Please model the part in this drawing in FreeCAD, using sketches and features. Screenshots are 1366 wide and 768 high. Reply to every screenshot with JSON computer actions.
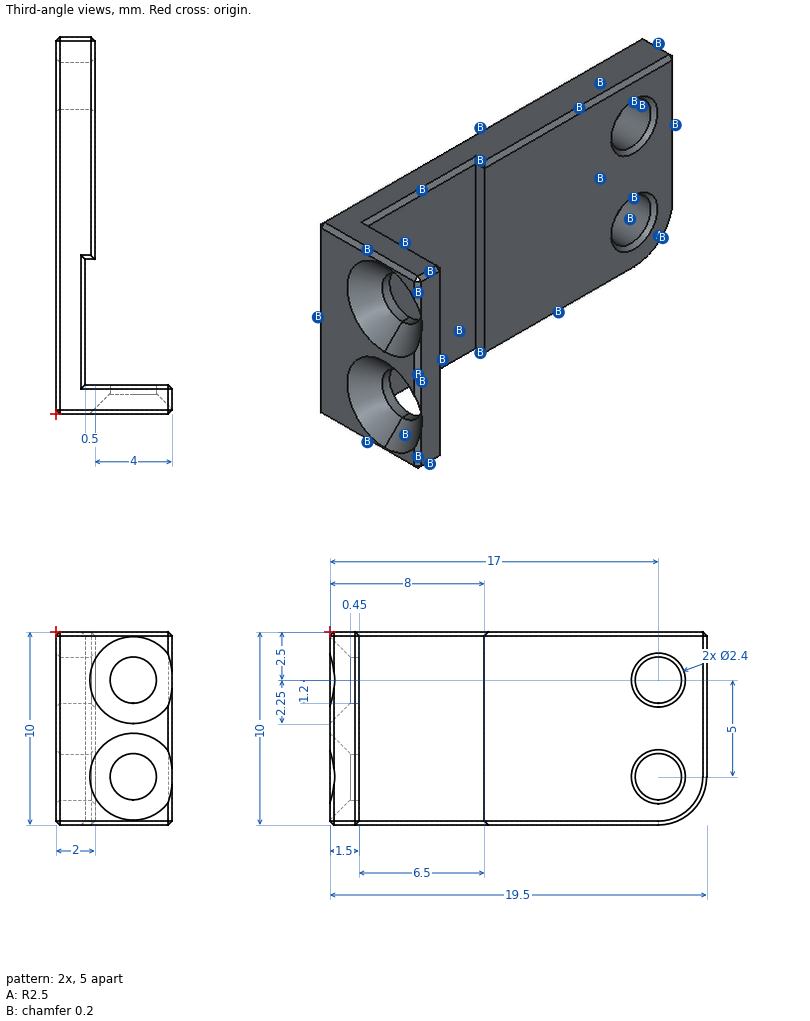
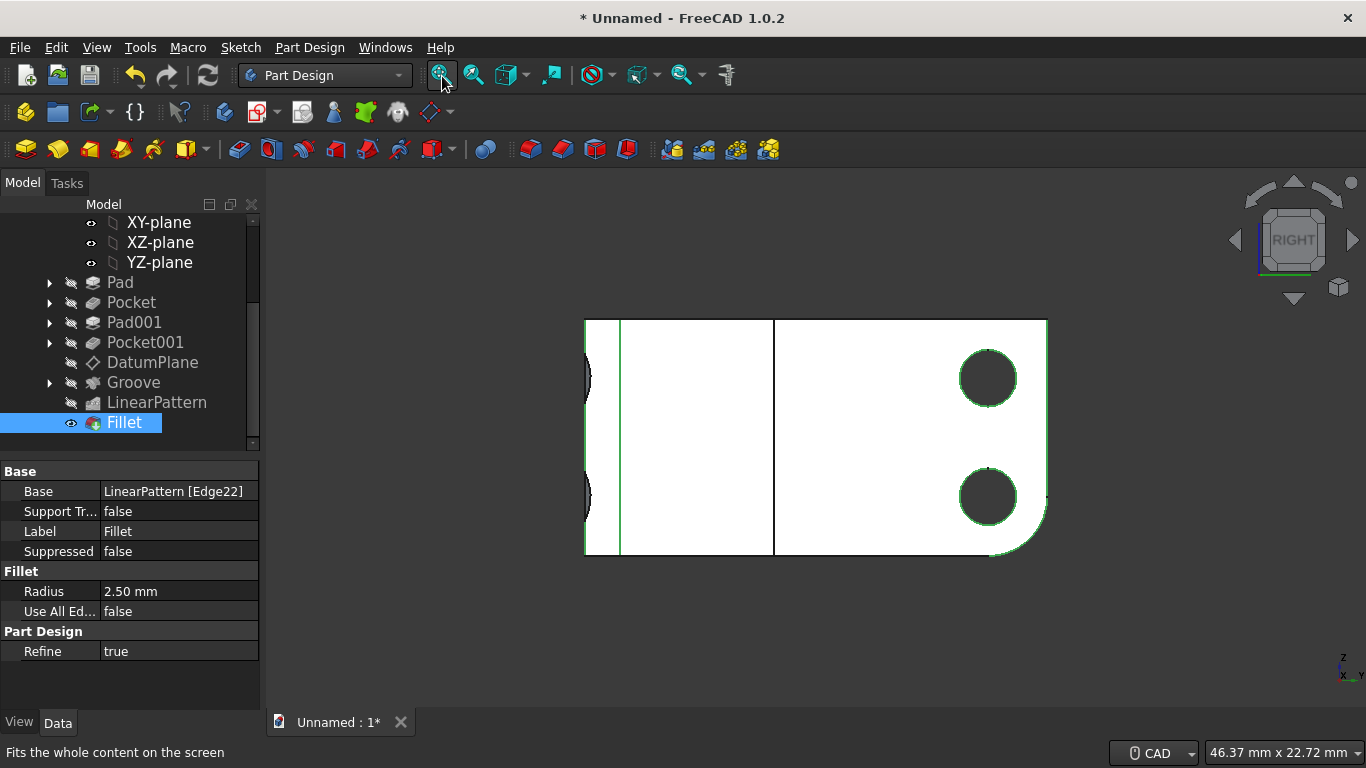
{"action": "left_click", "coordinate": [602, 555], "text": "ctrl"}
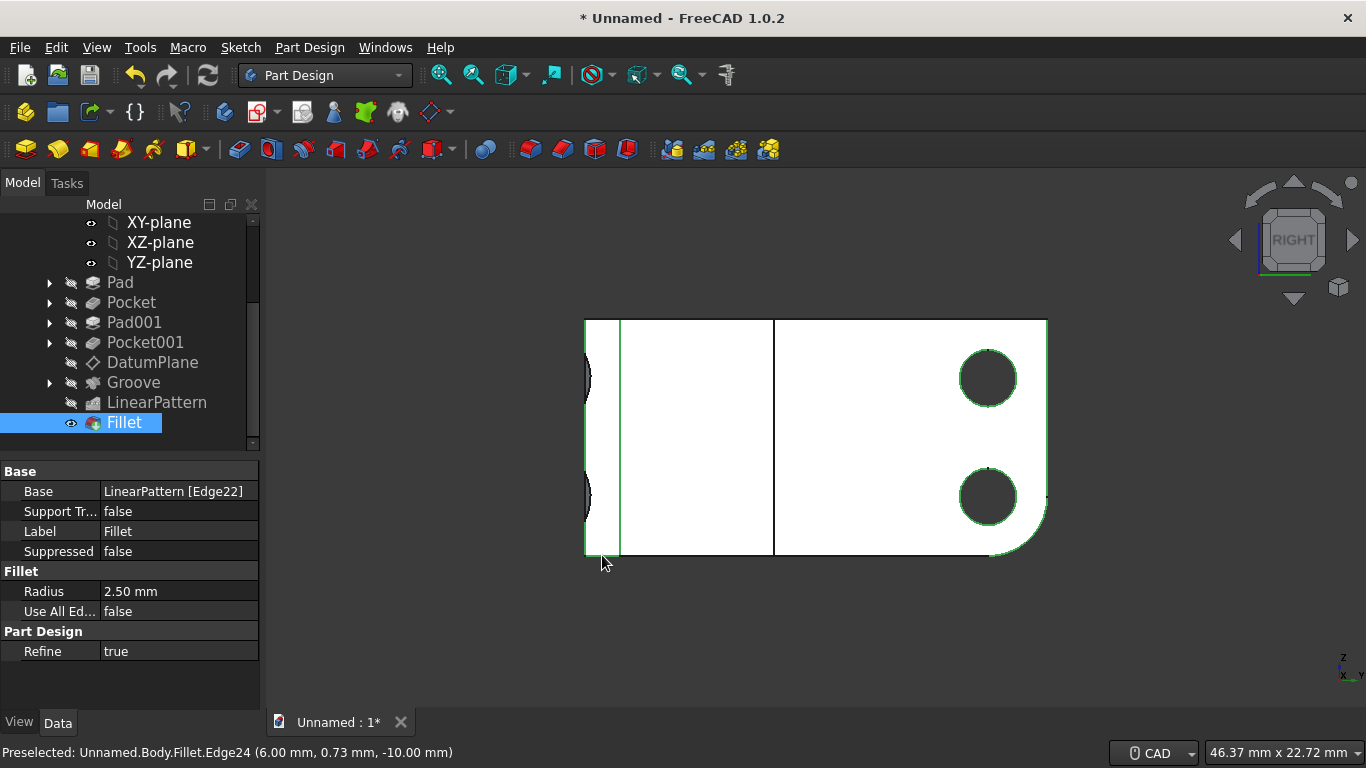
{"action": "left_click", "coordinate": [881, 555], "text": "ctrl"}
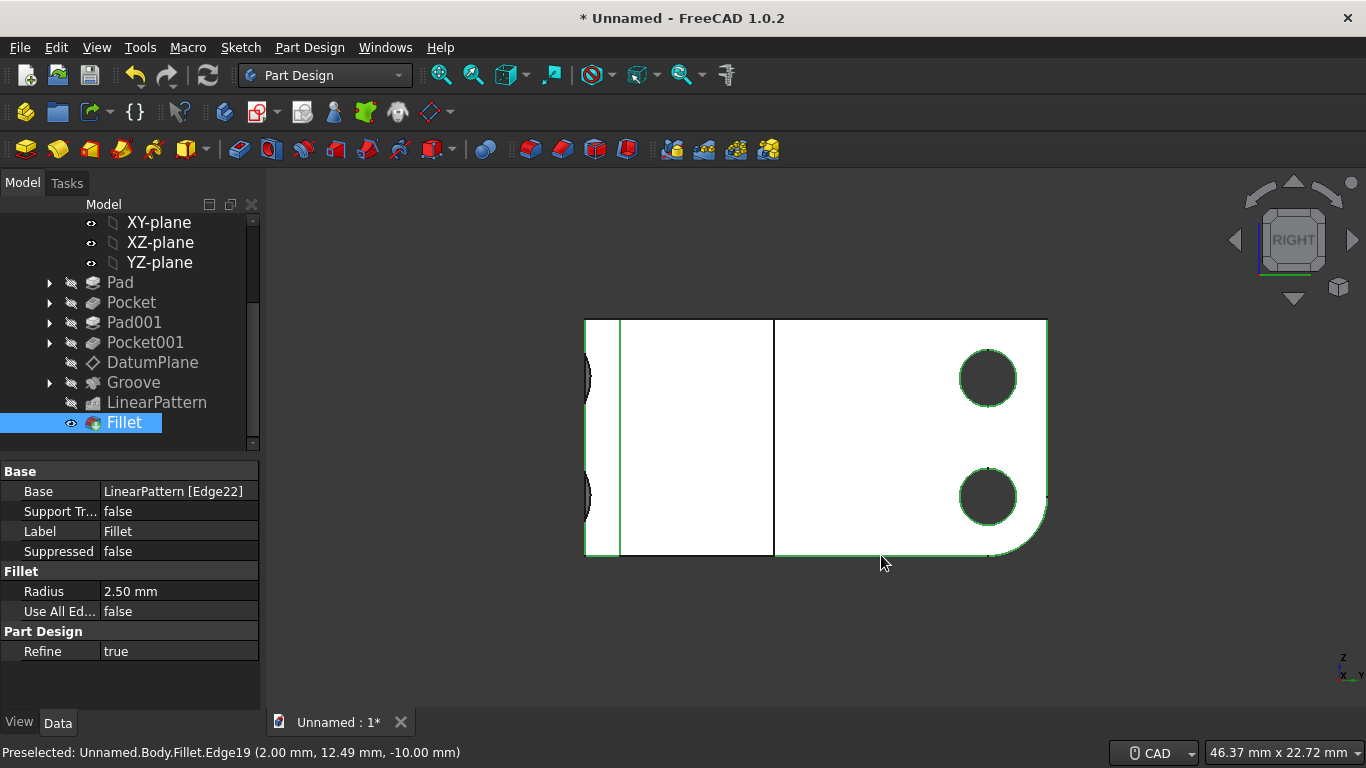
{"action": "left_click", "coordinate": [697, 555], "text": "ctrl"}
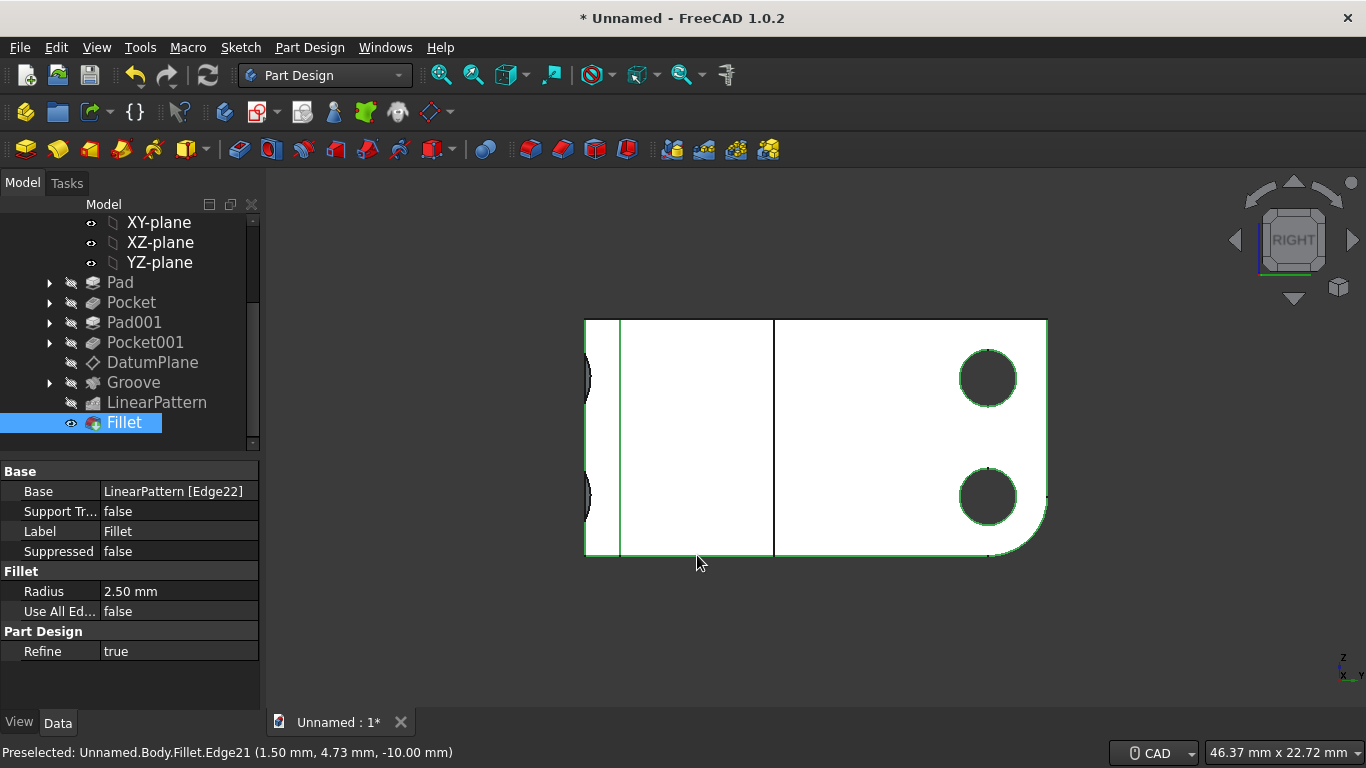
{"action": "key", "text": "5"}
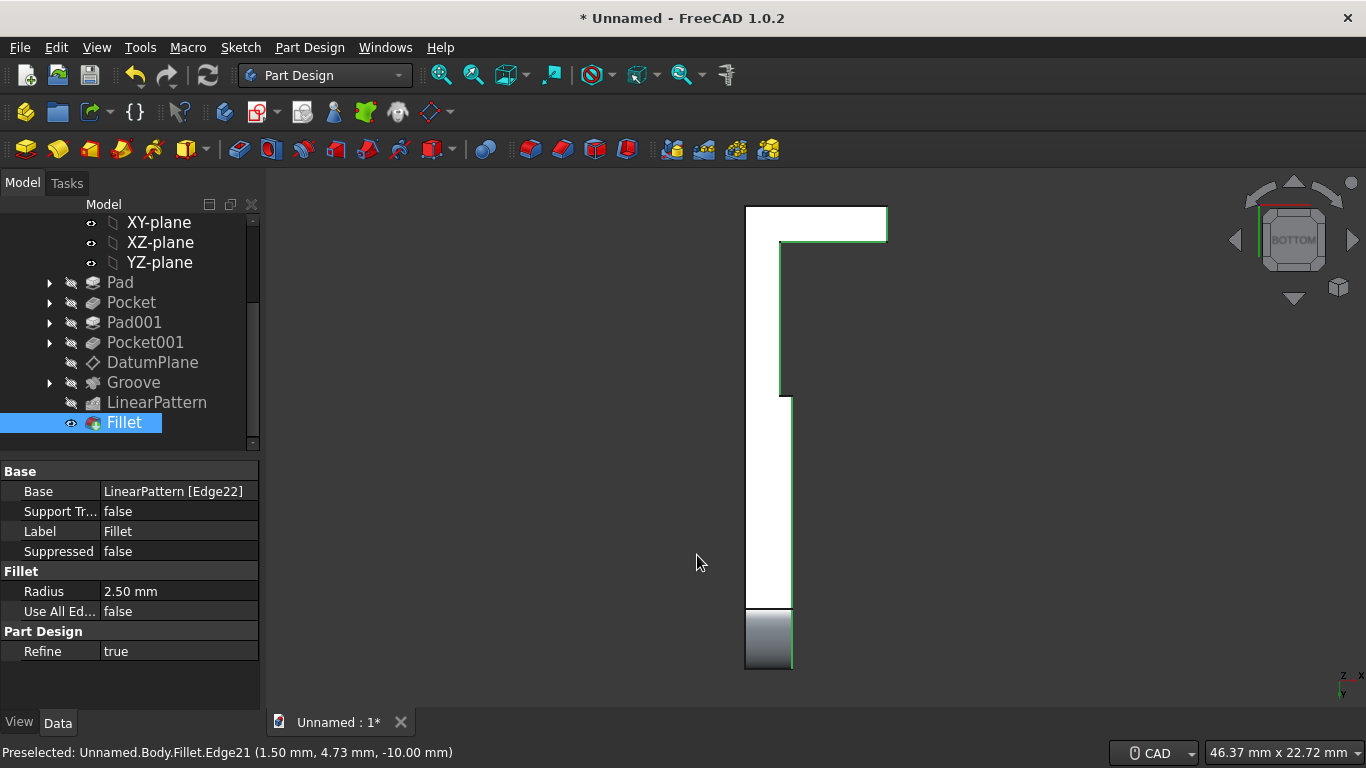
{"action": "left_click", "coordinate": [816, 205], "text": "ctrl"}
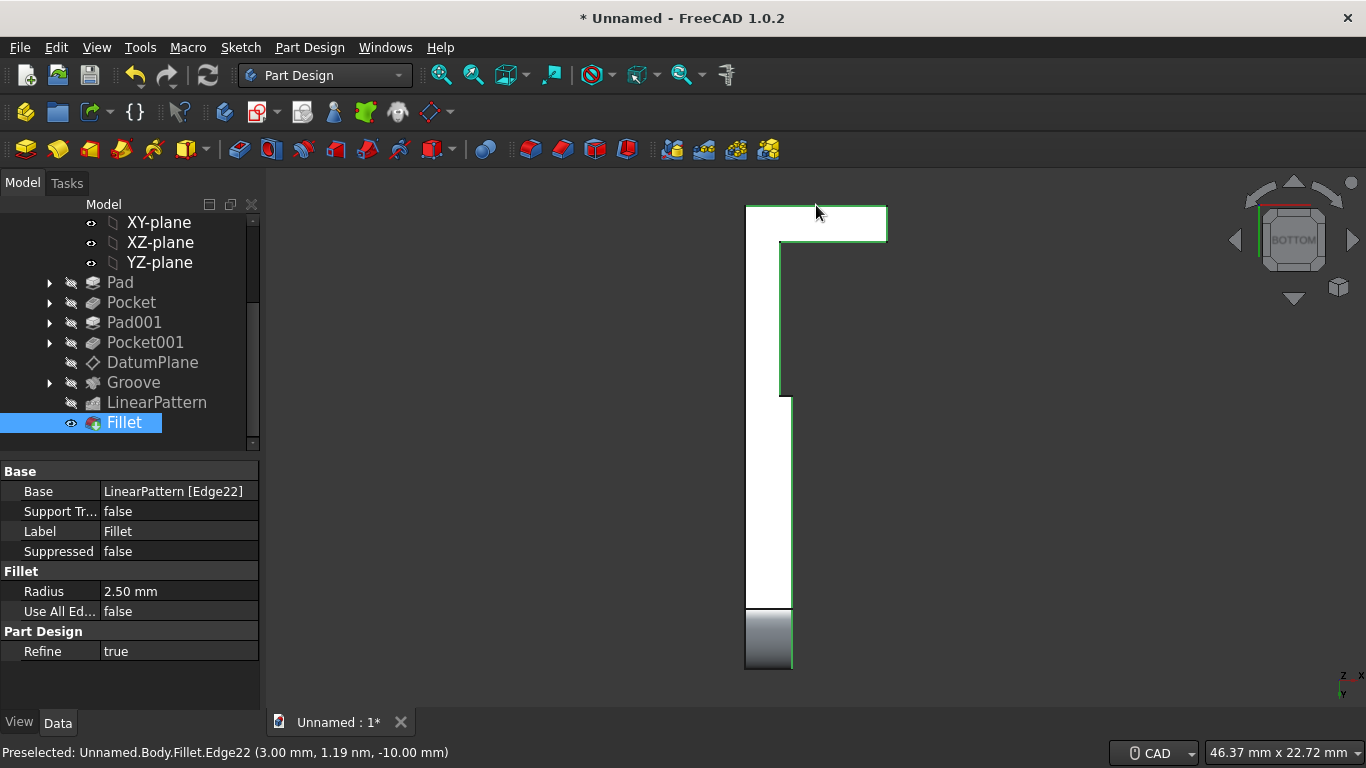
{"action": "key", "text": "4"}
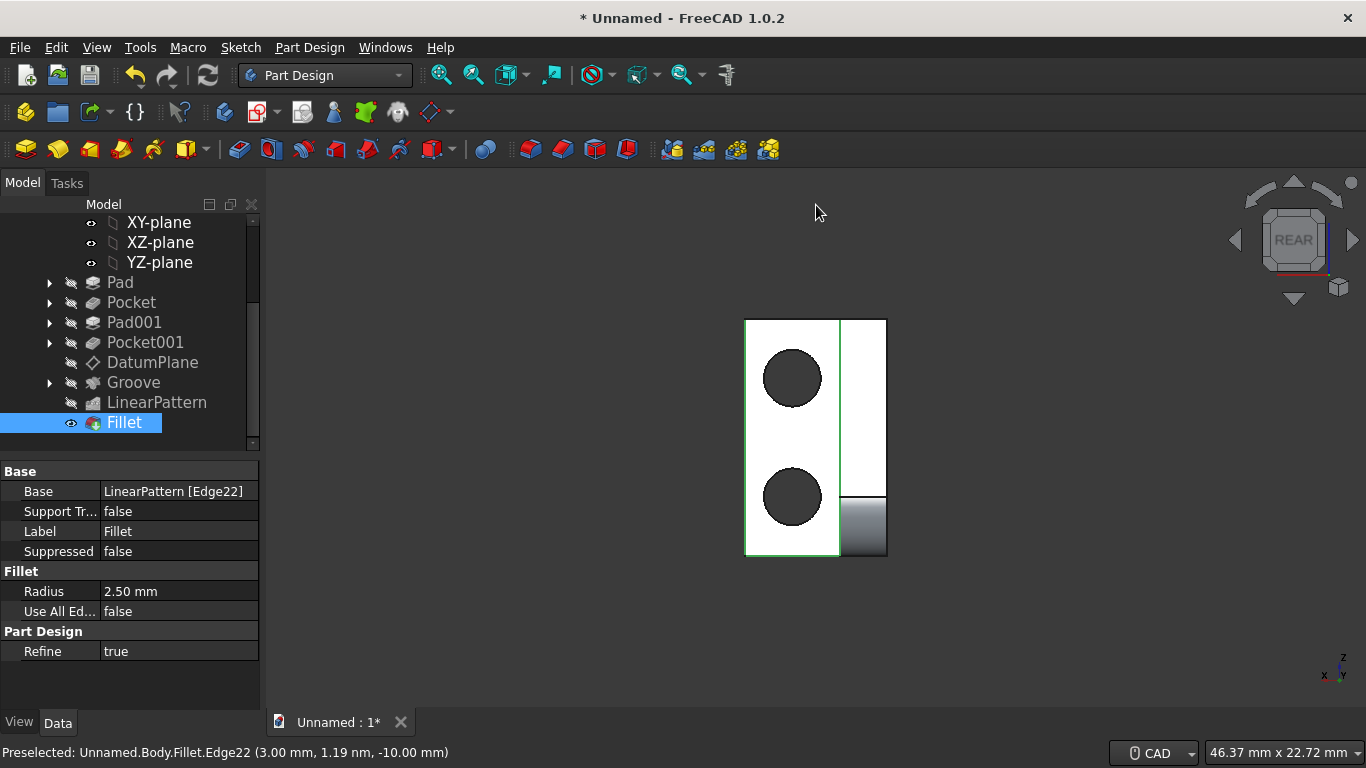
{"action": "left_click", "coordinate": [442, 76]}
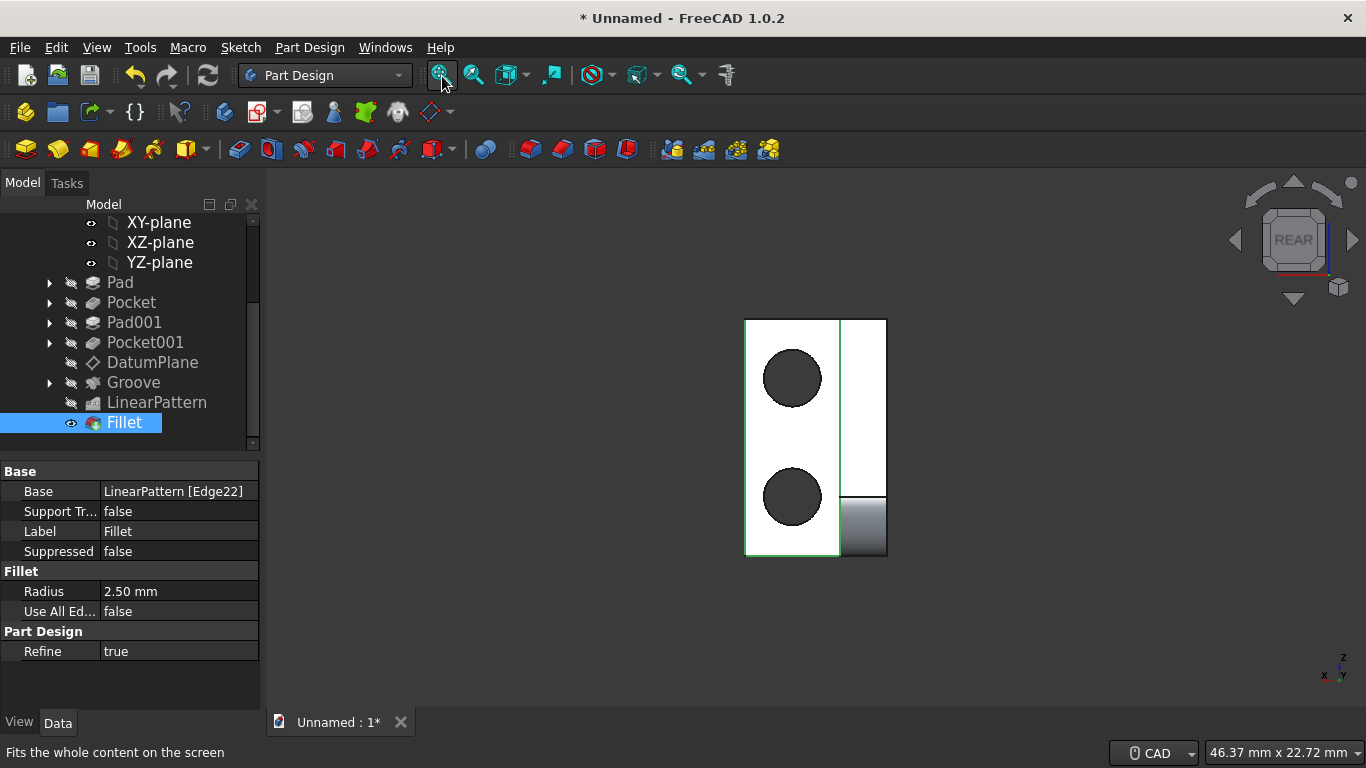
{"action": "key", "text": "6"}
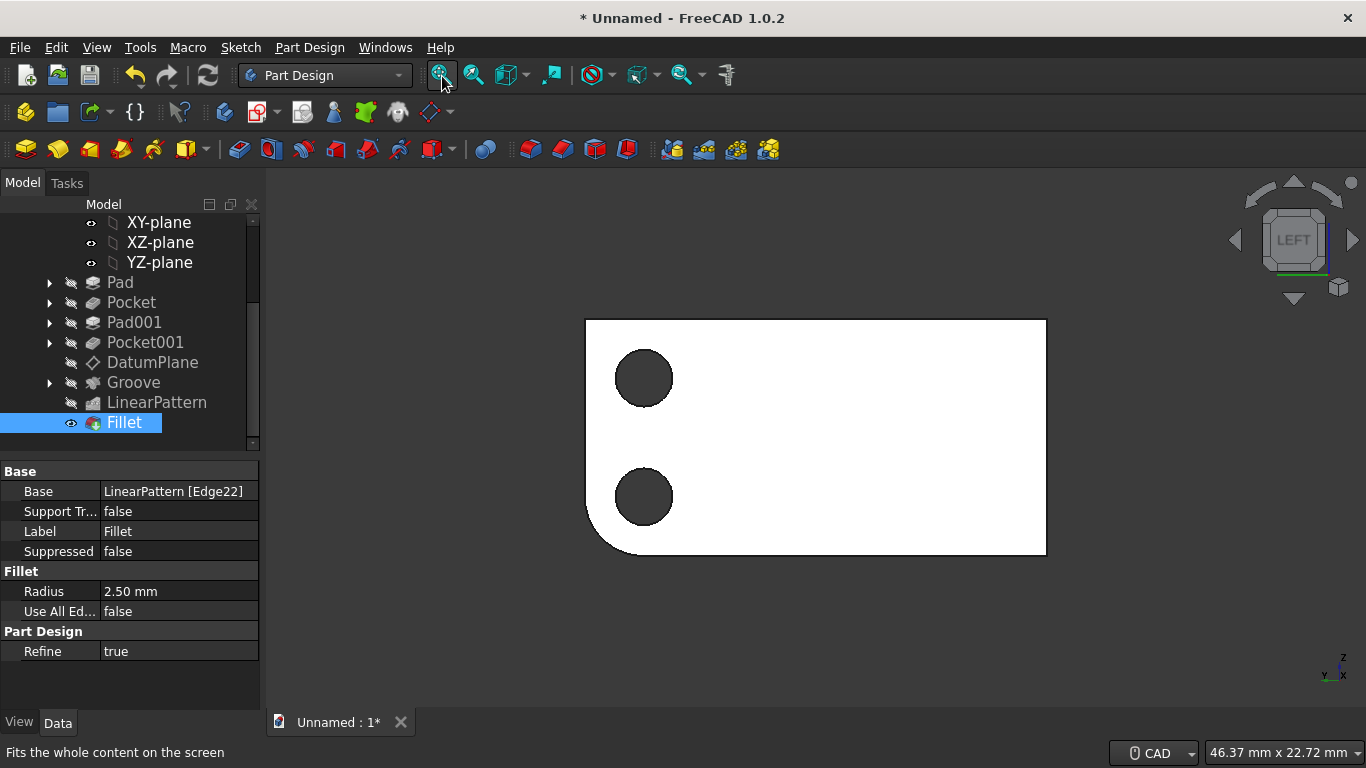
{"action": "left_click", "coordinate": [442, 76]}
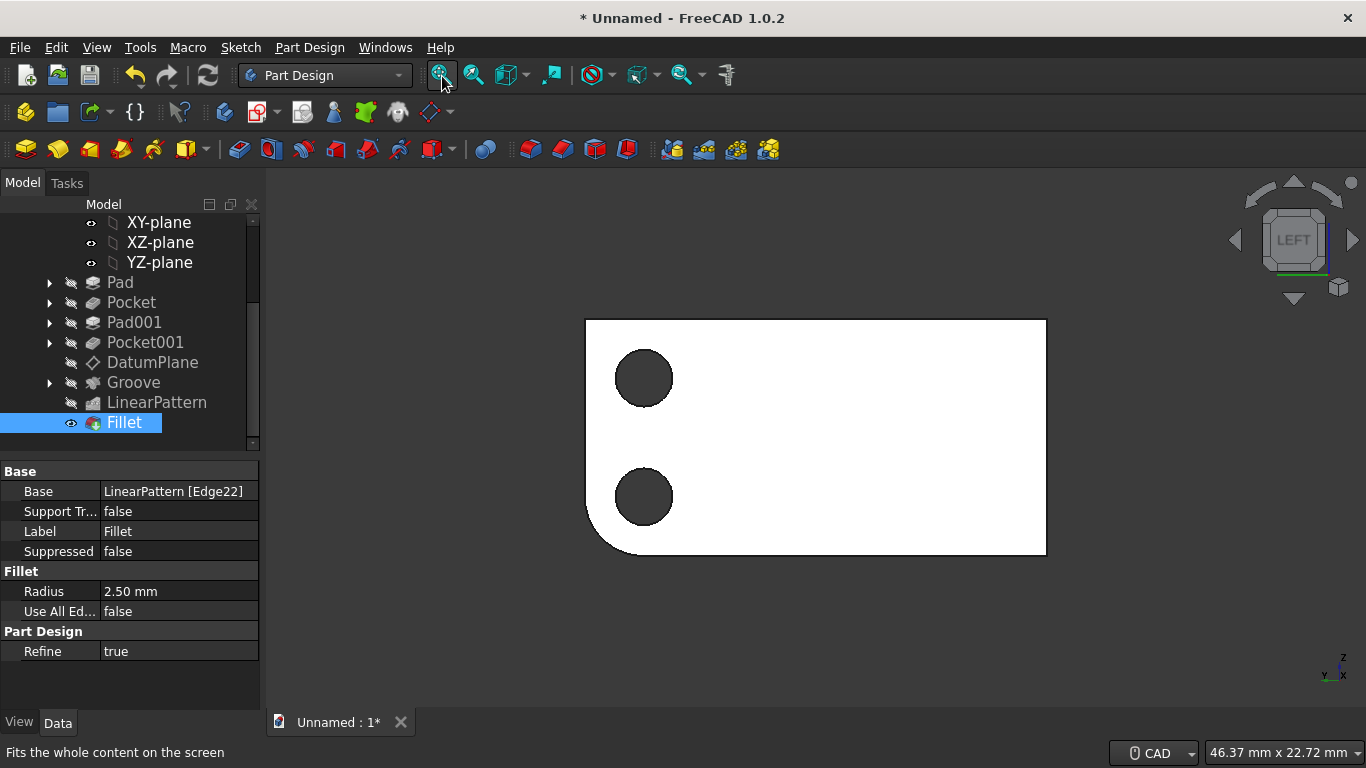
{"action": "left_click", "coordinate": [882, 437], "text": "ctrl"}